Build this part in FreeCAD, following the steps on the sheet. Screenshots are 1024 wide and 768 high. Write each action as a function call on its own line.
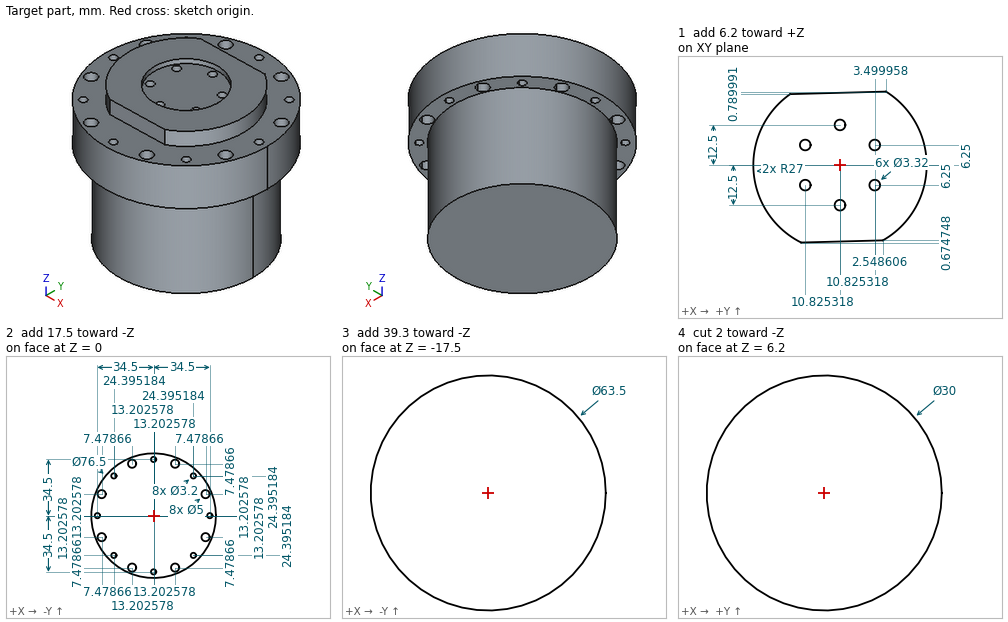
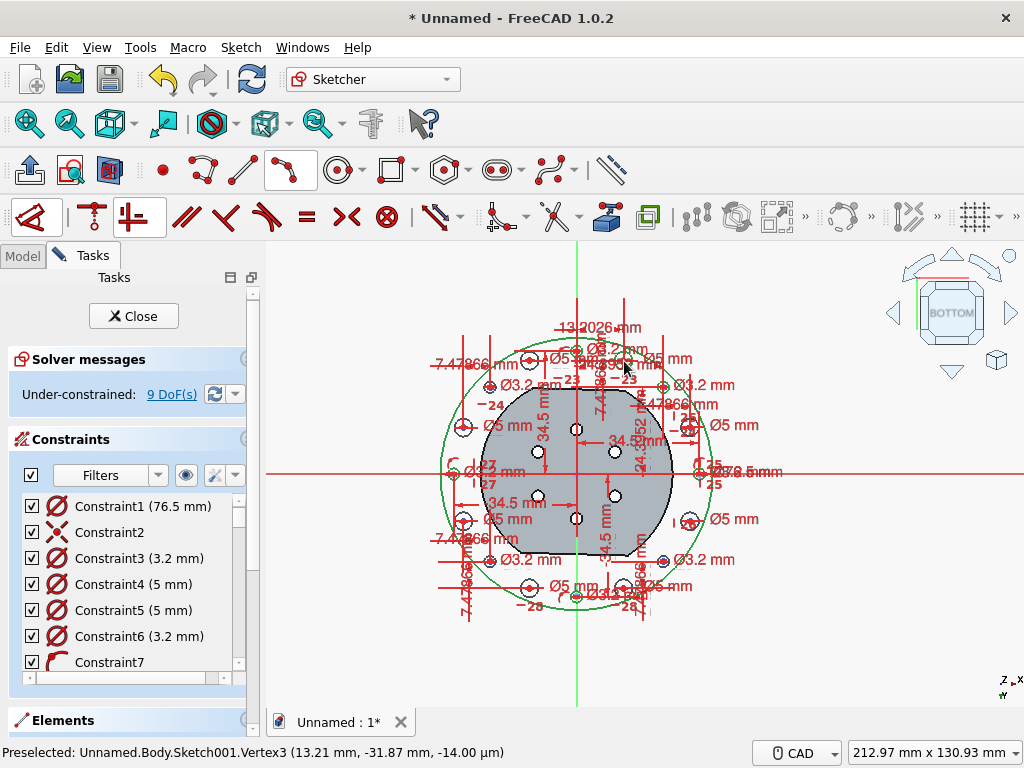
click(690, 427)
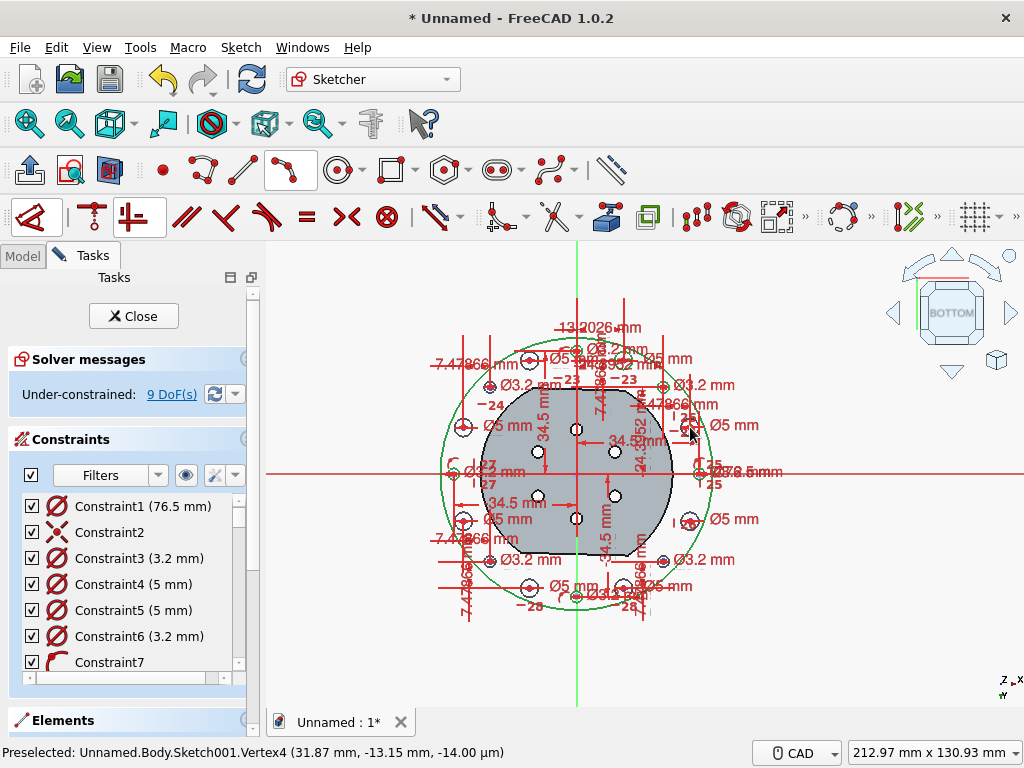
click(56, 218)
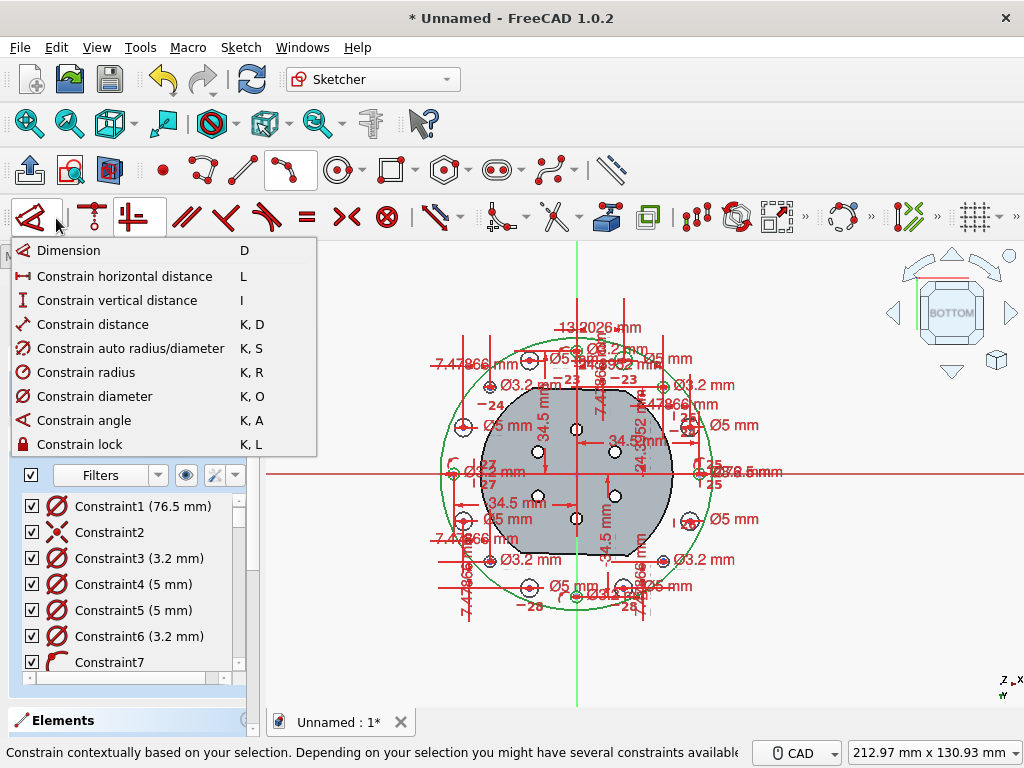
click(164, 300)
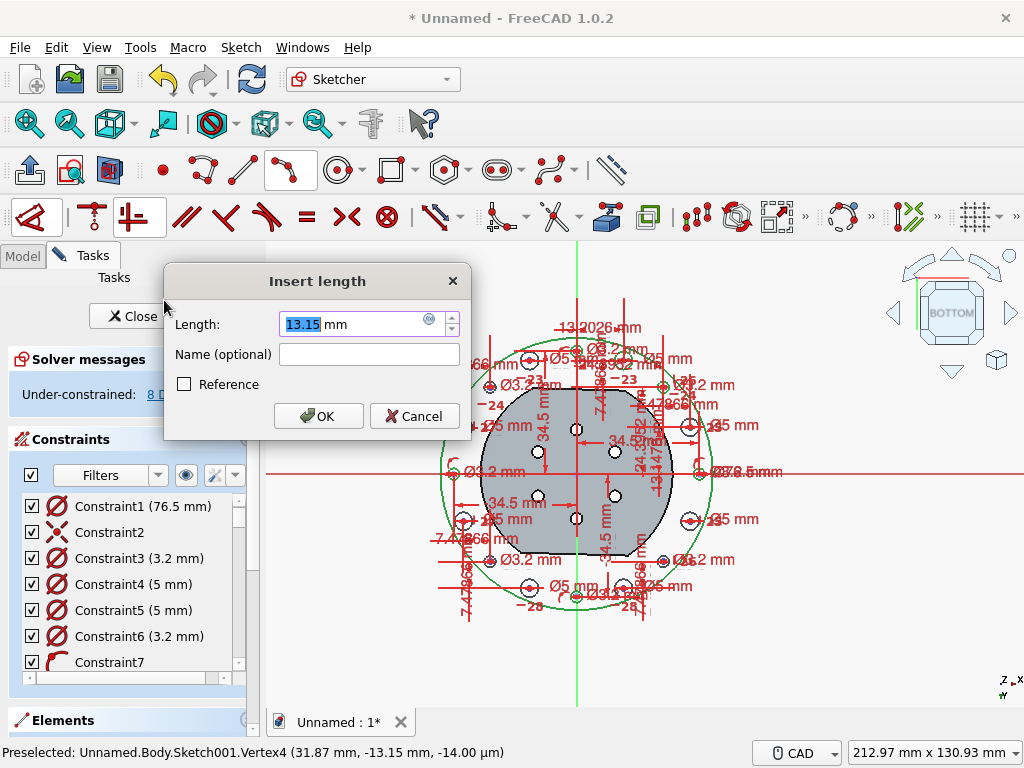
text(13.202578)
key(Return)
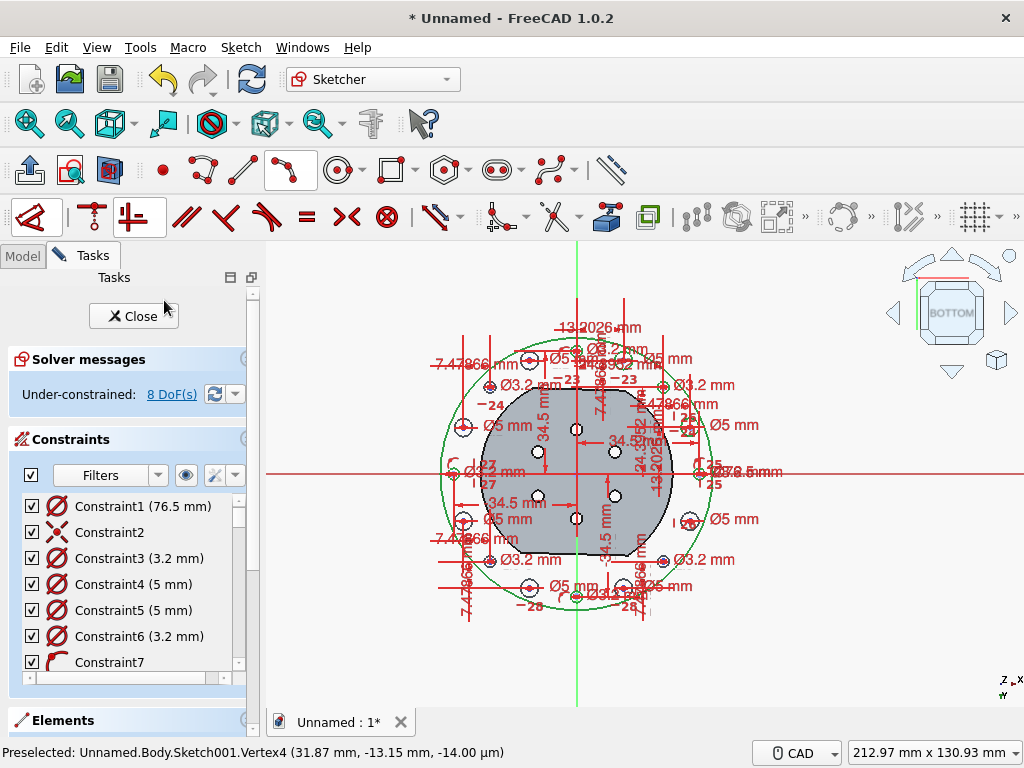
click(530, 361)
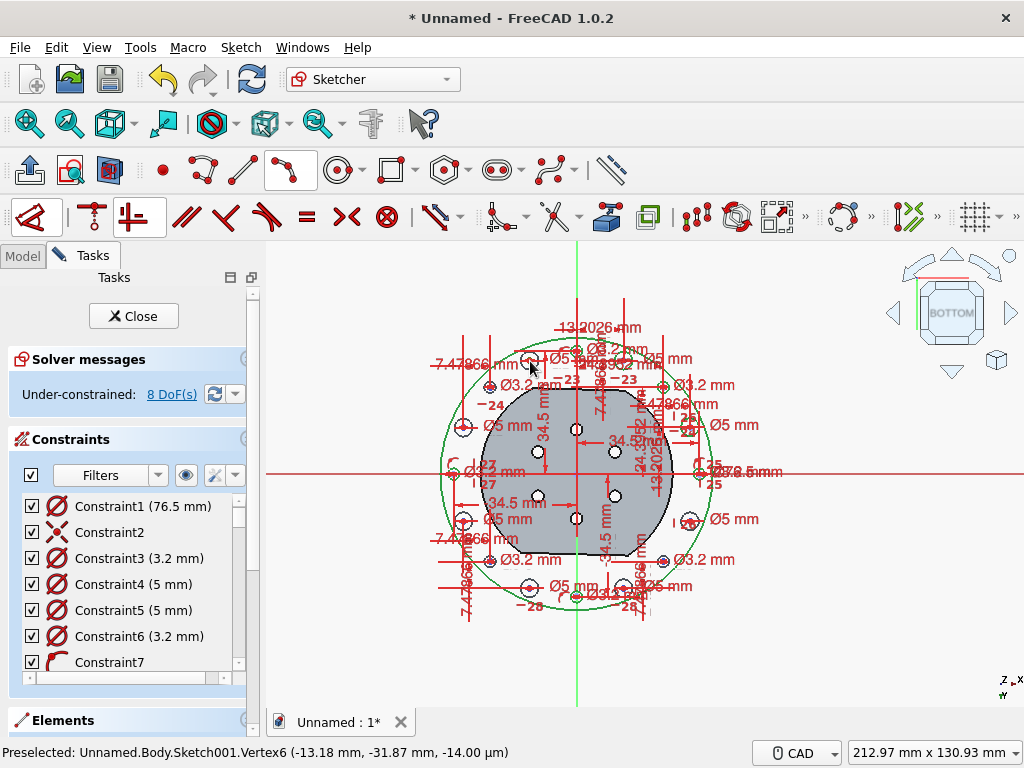
key(l)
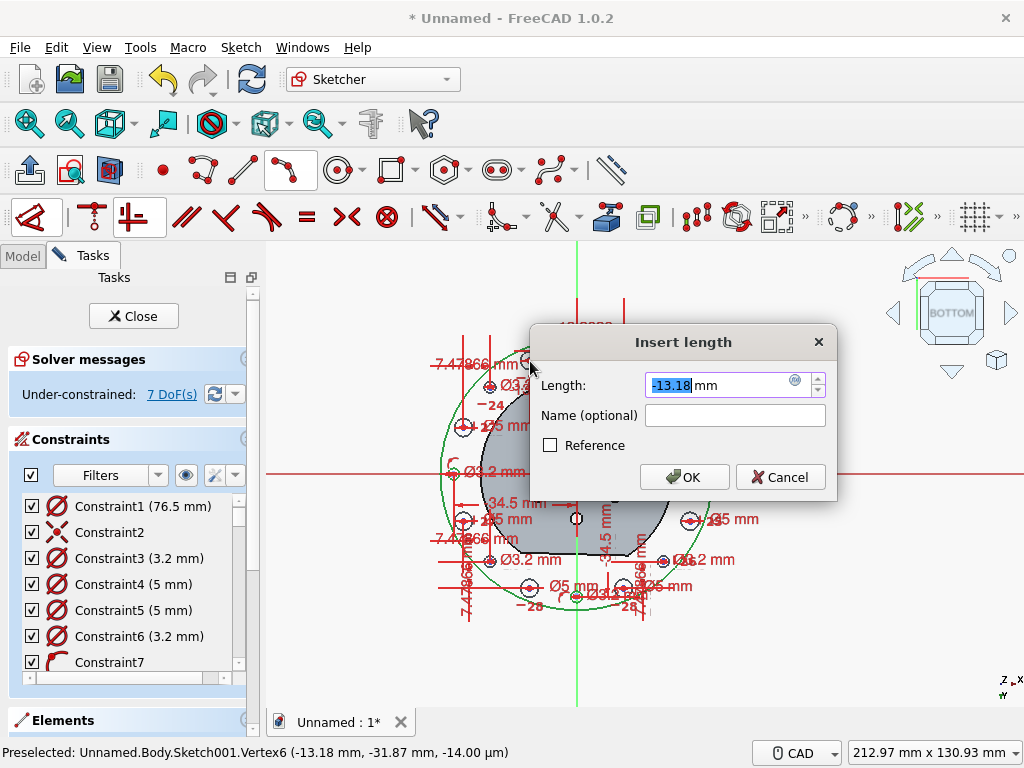
text(-13.202578)
key(Return)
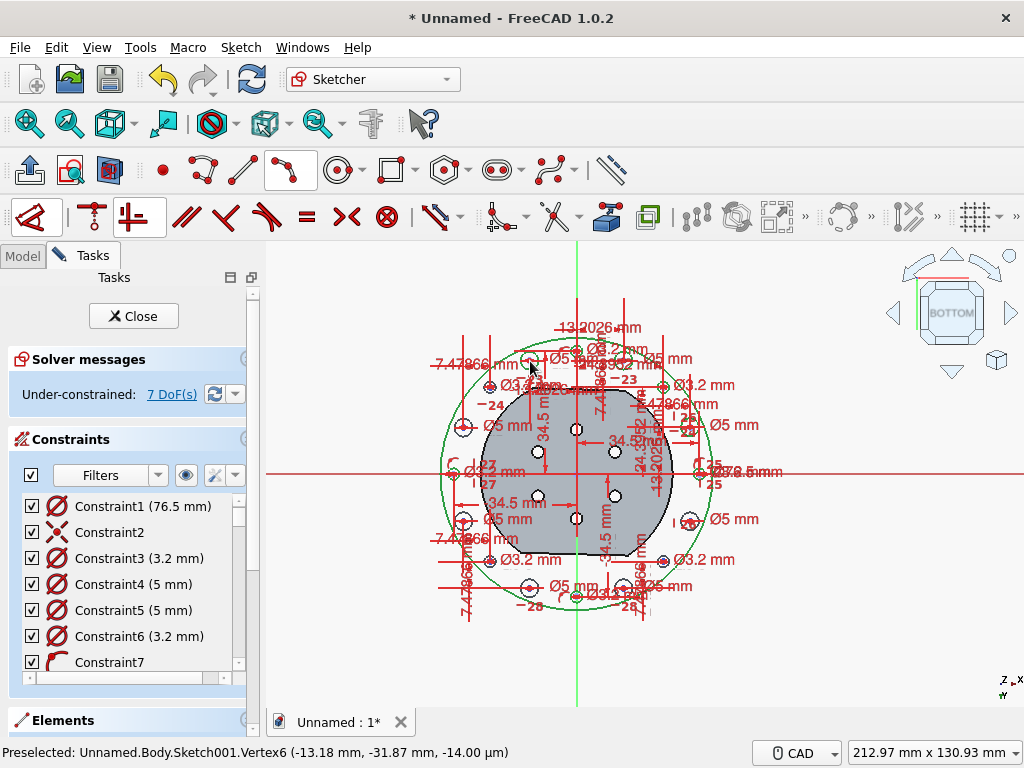
click(490, 387)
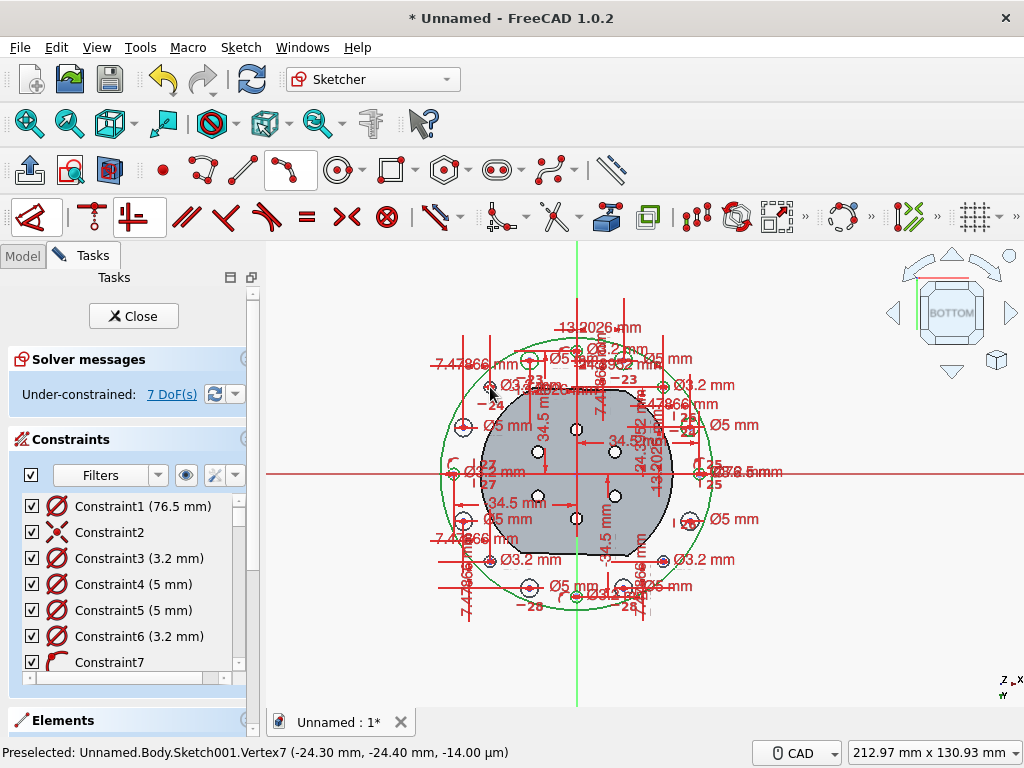
key(l)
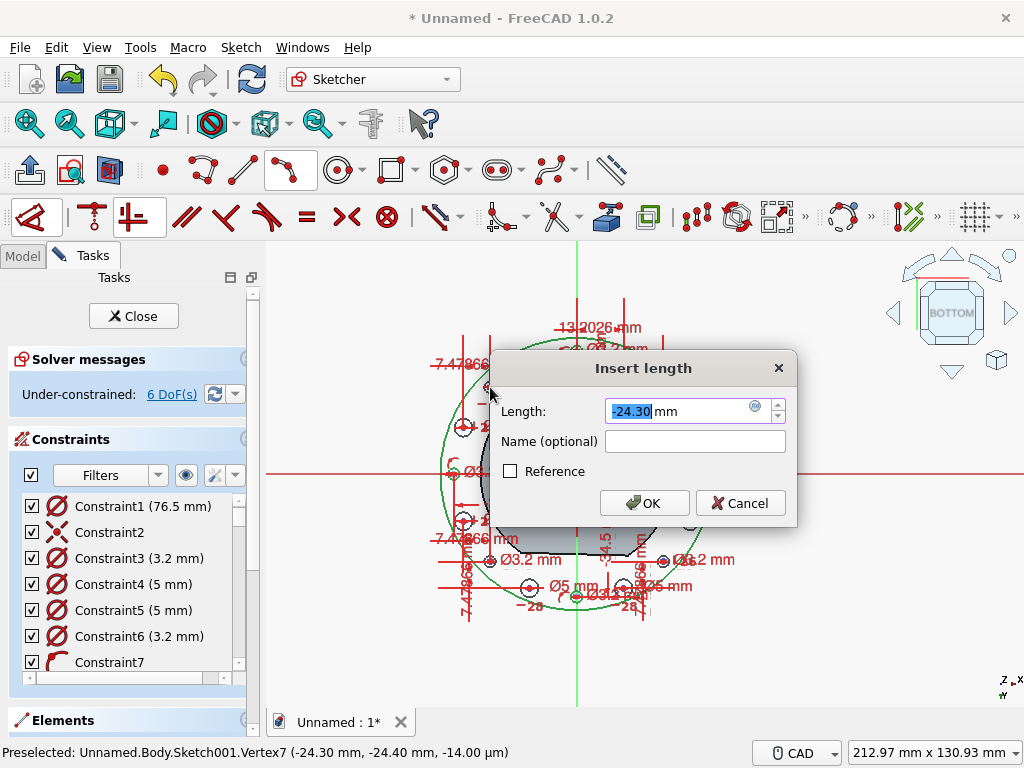
text(-24.395184)
key(Return)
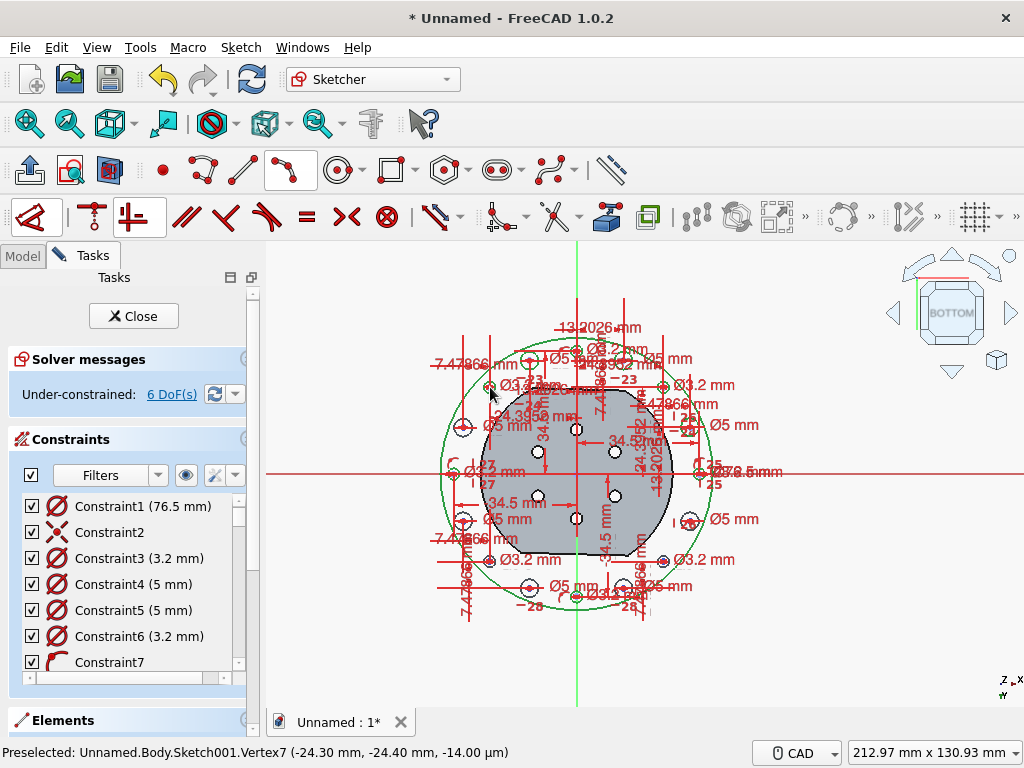
click(463, 428)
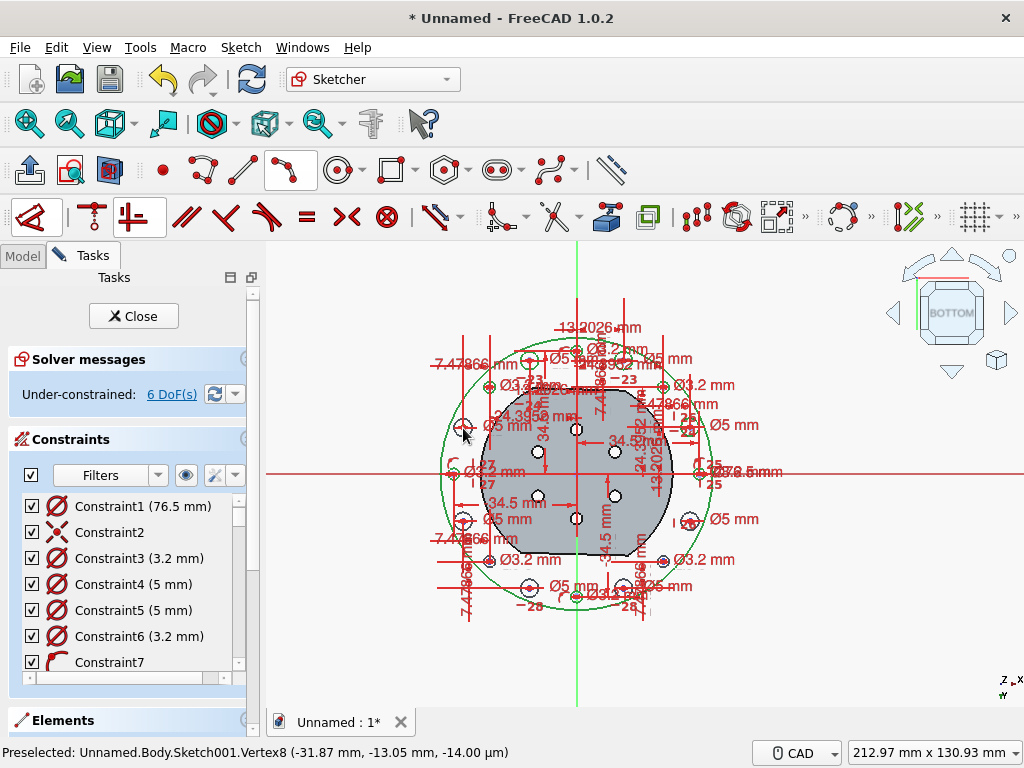
key(i)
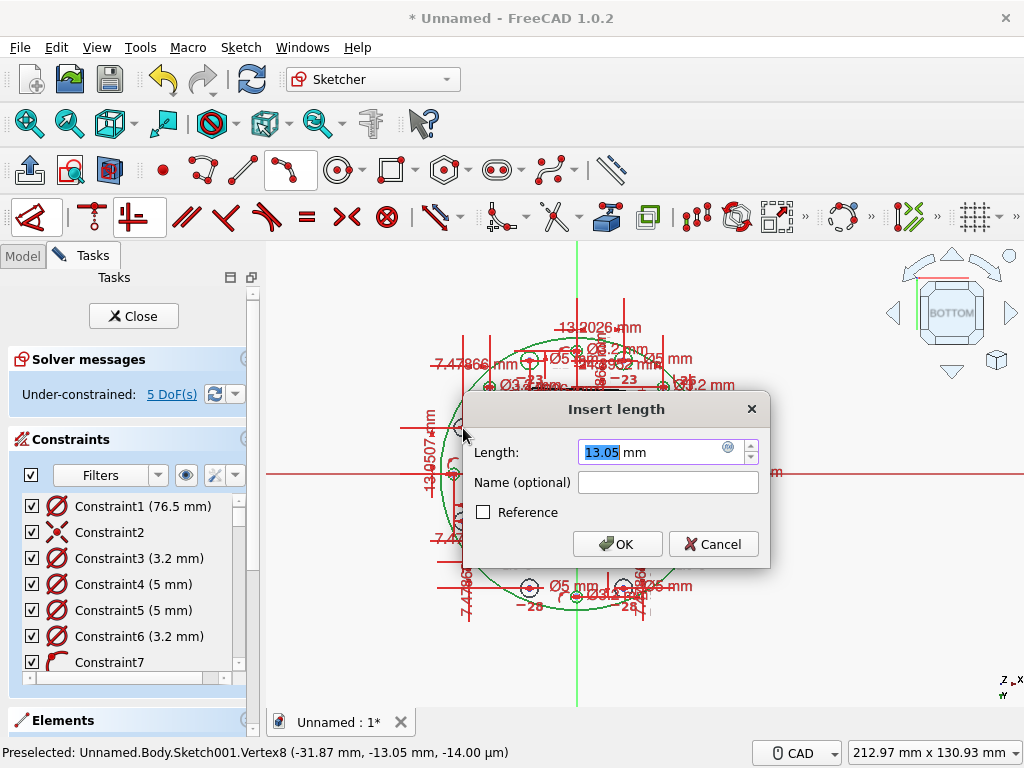
text(13.202578)
key(Return)